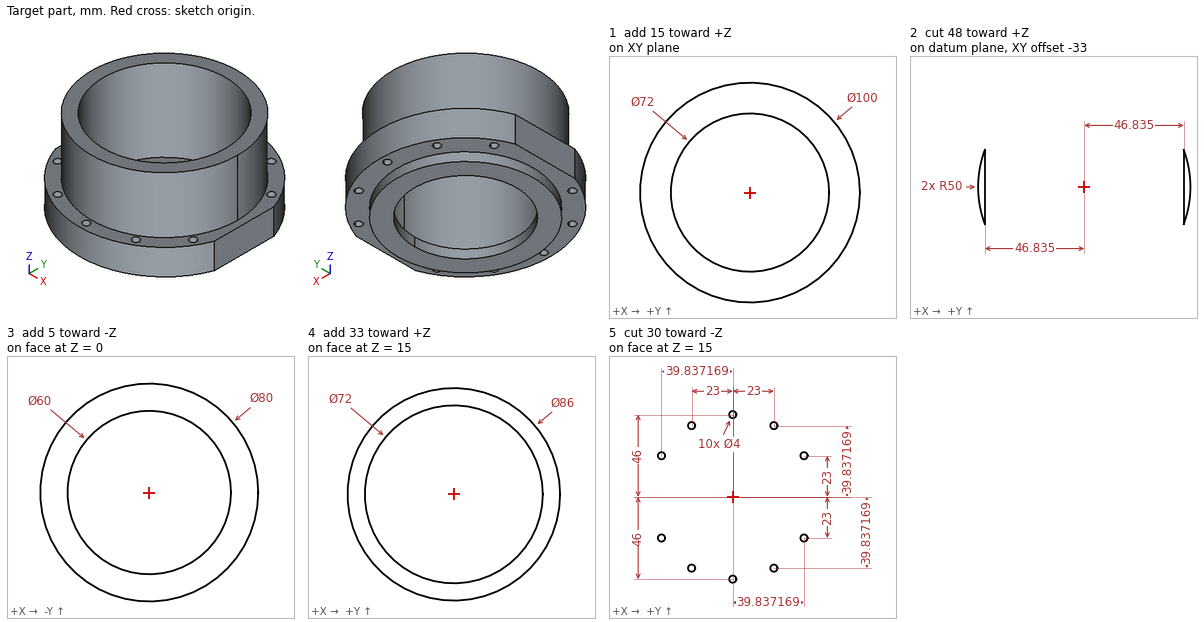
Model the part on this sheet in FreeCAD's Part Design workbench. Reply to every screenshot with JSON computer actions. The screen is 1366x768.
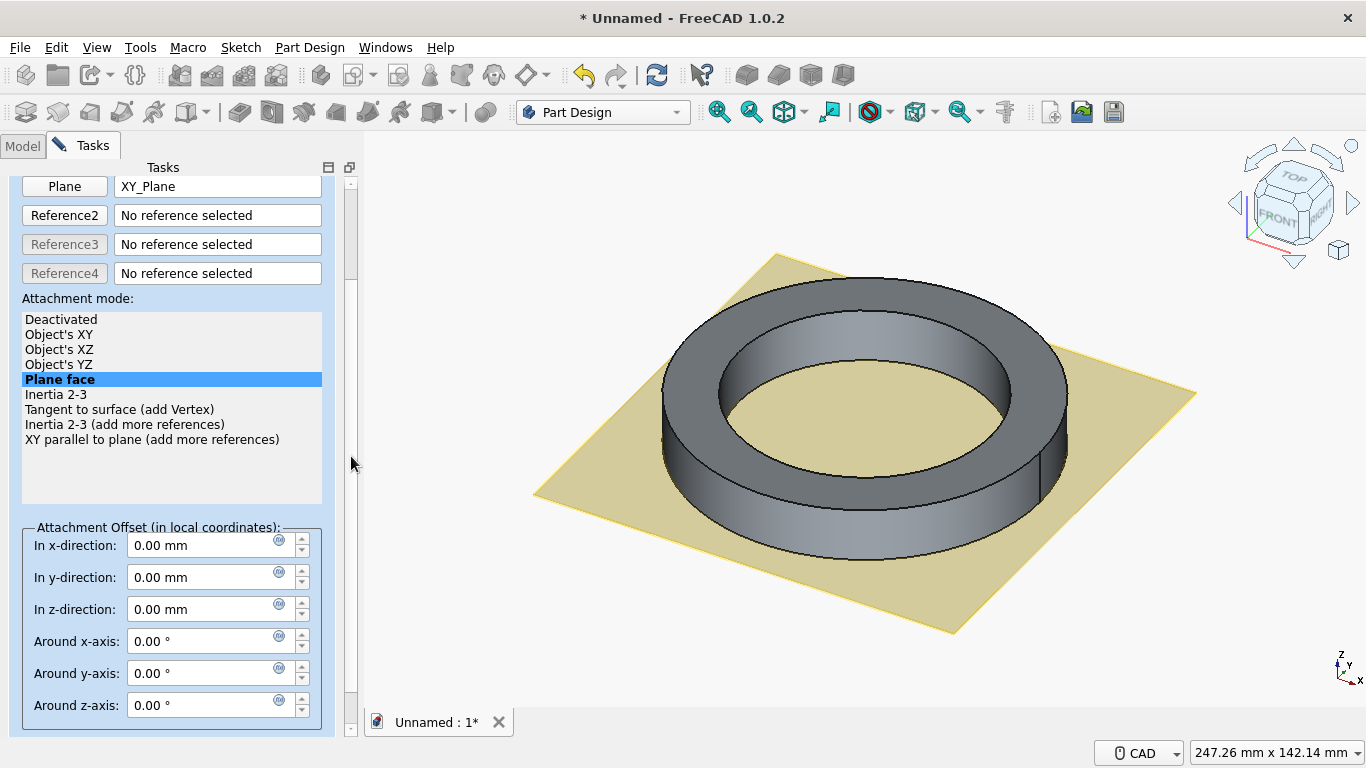
{"action": "triple_click", "coordinate": [210, 609]}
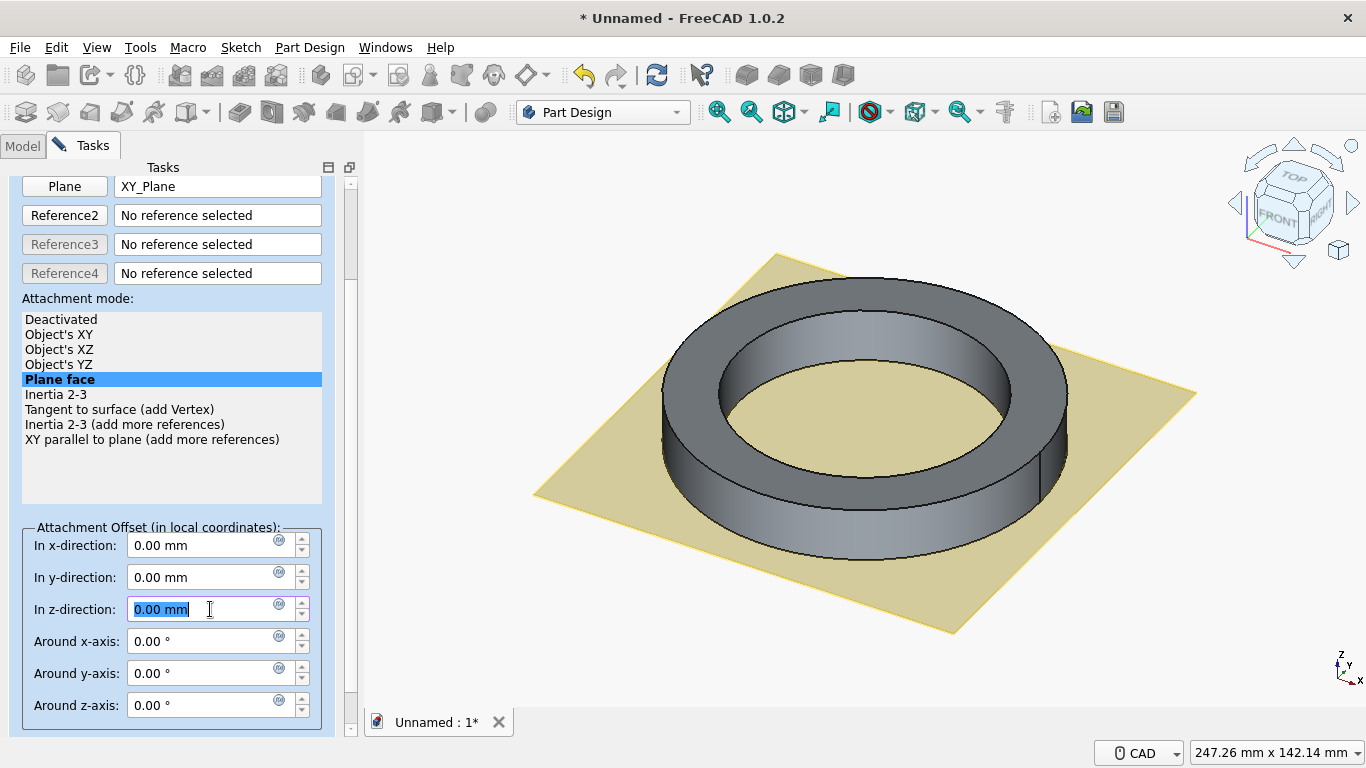
{"action": "type", "text": "-33"}
{"action": "key", "text": "Tab"}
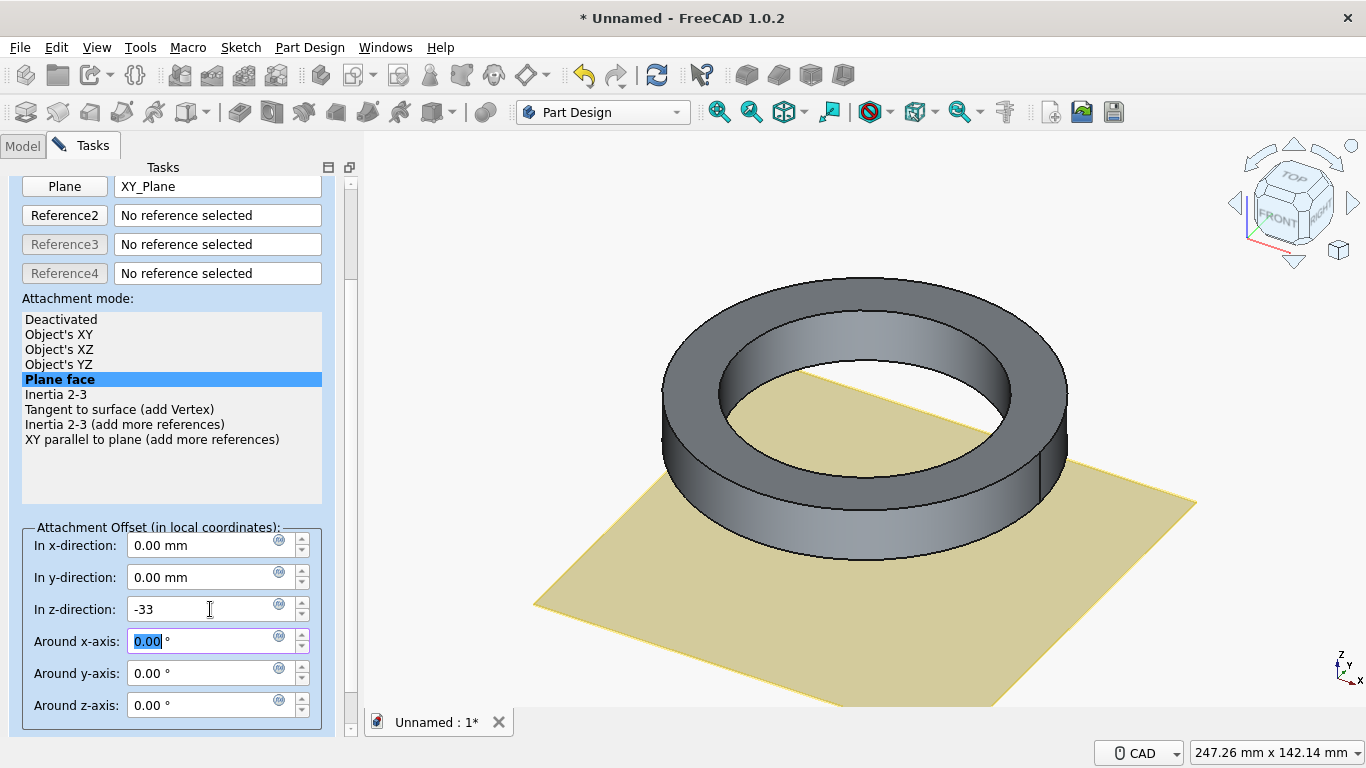
{"action": "scroll", "coordinate": [351, 456], "scroll_direction": "up", "scroll_amount": 3}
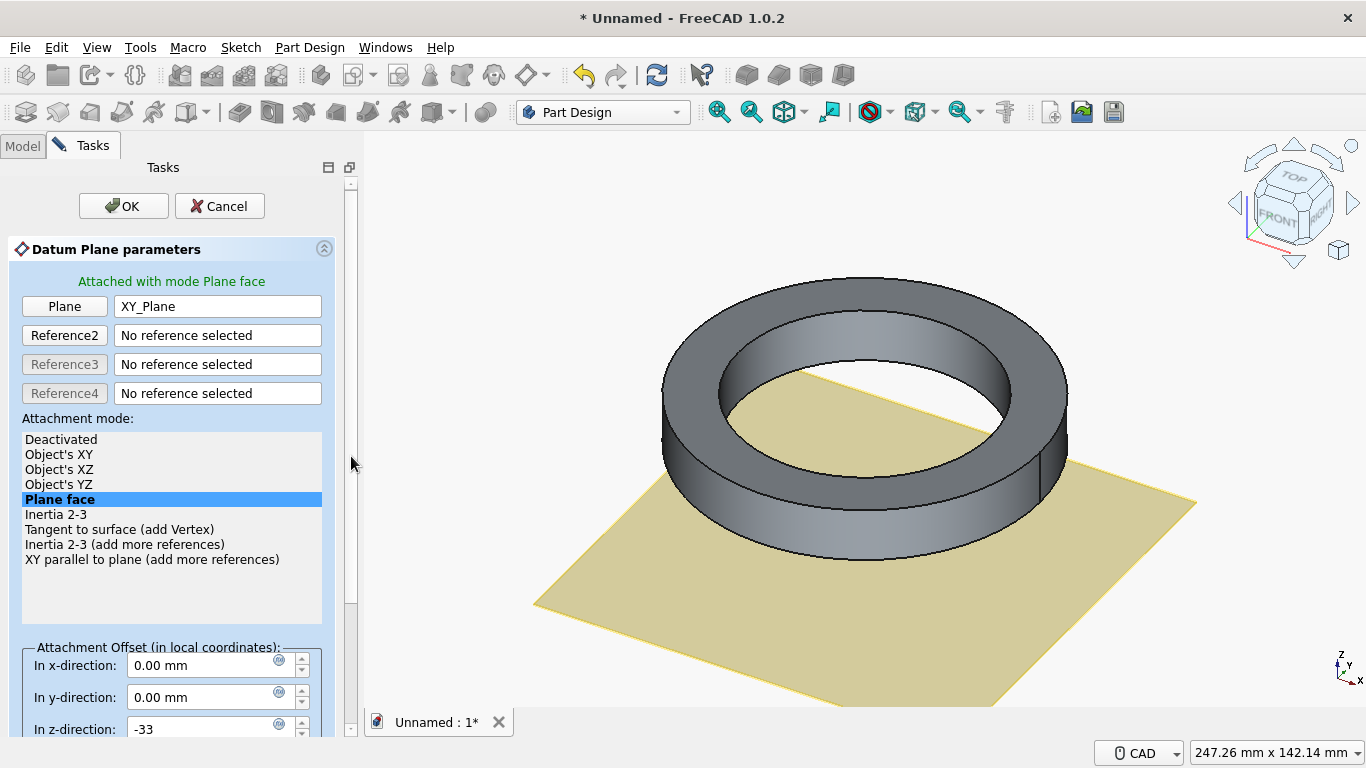
{"action": "left_click", "coordinate": [124, 206]}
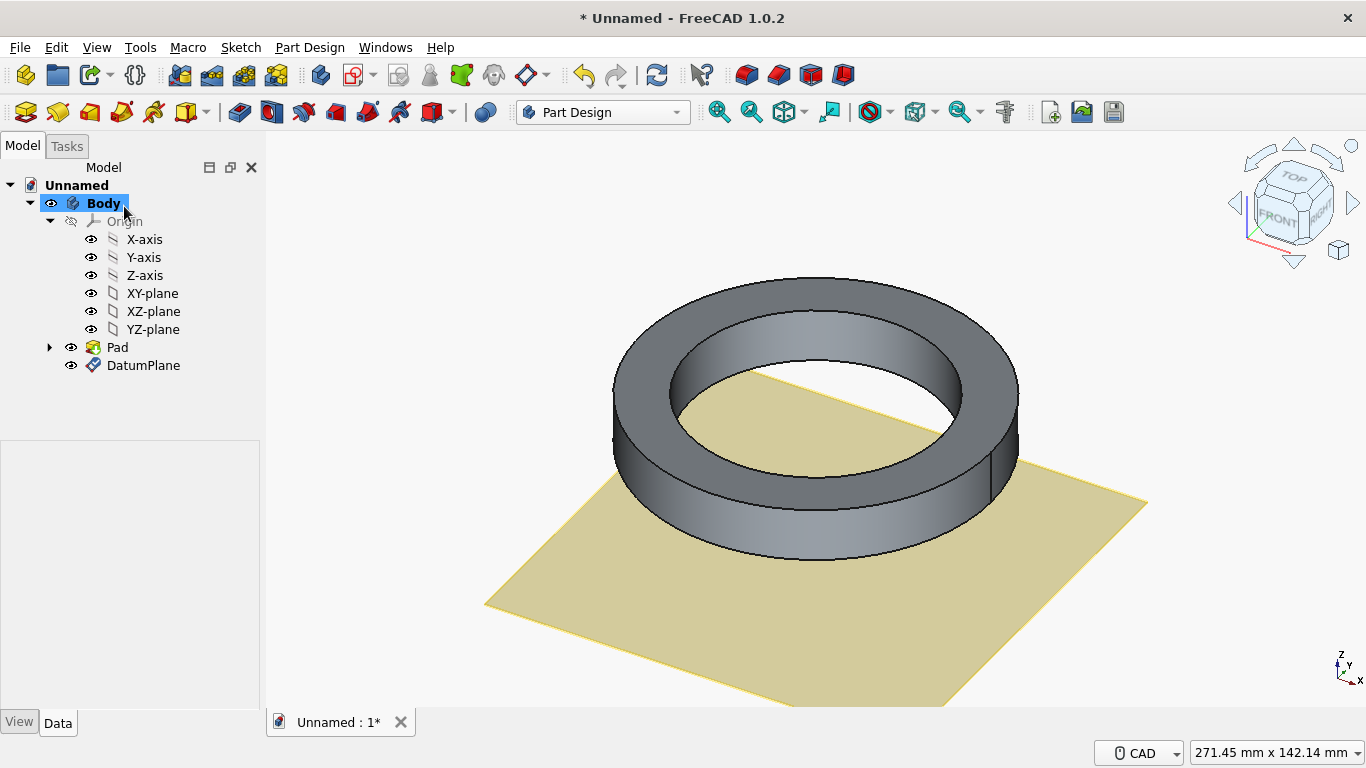
{"action": "left_click", "coordinate": [116, 365]}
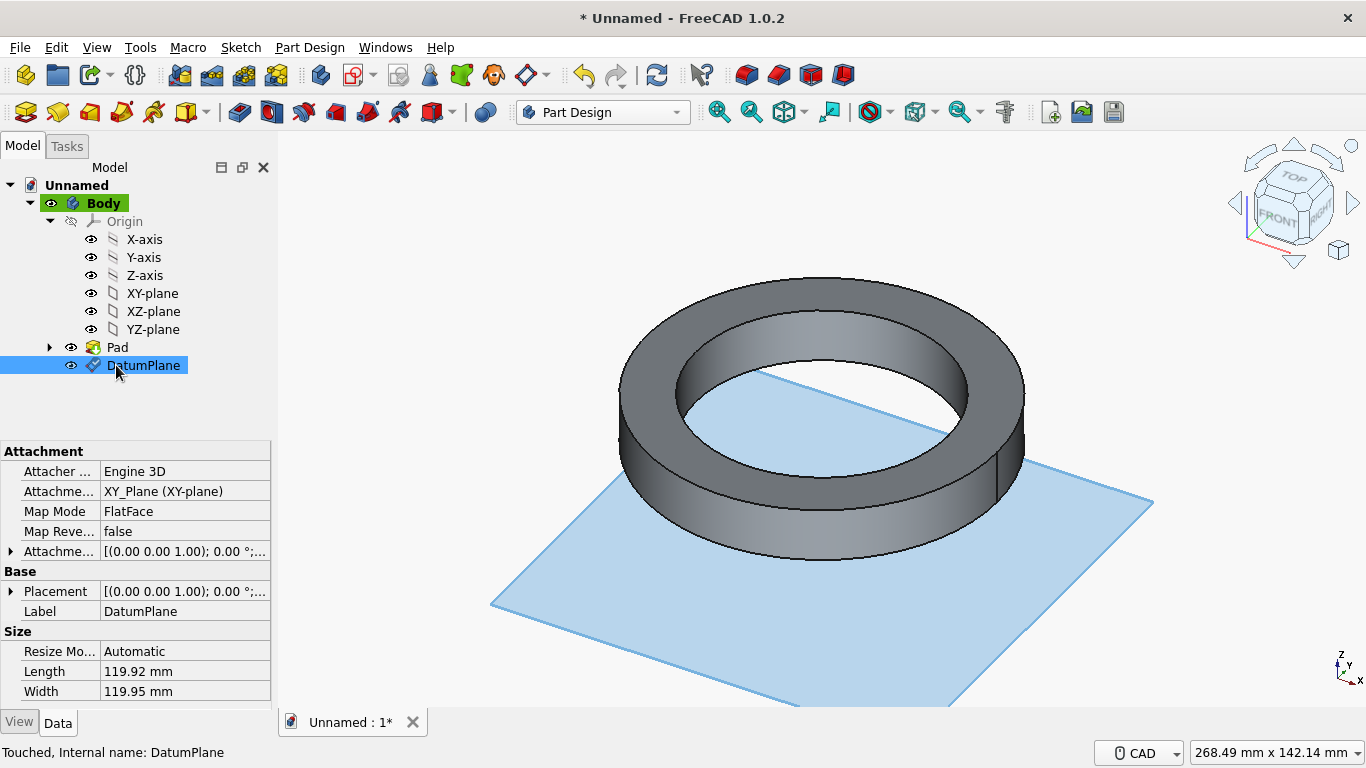
{"action": "left_click", "coordinate": [354, 76]}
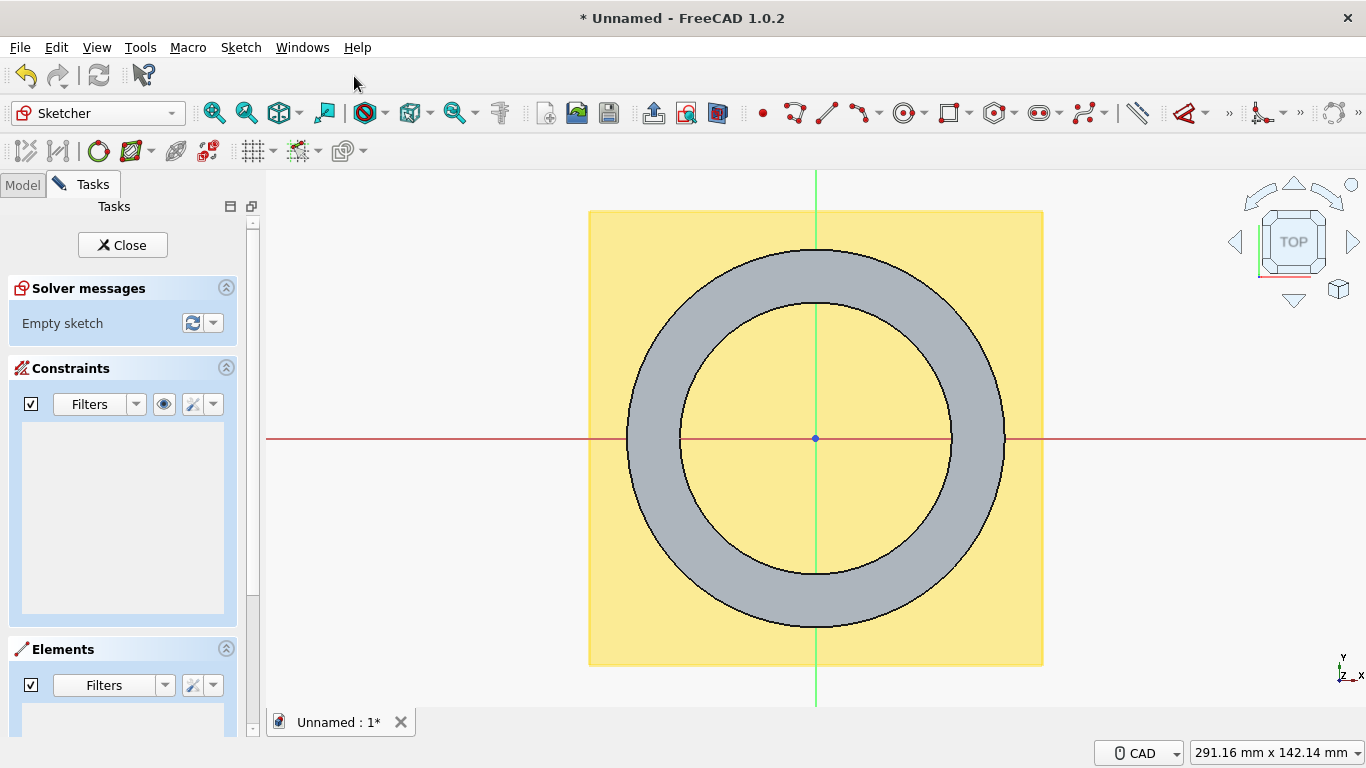
{"action": "left_click", "coordinate": [718, 114]}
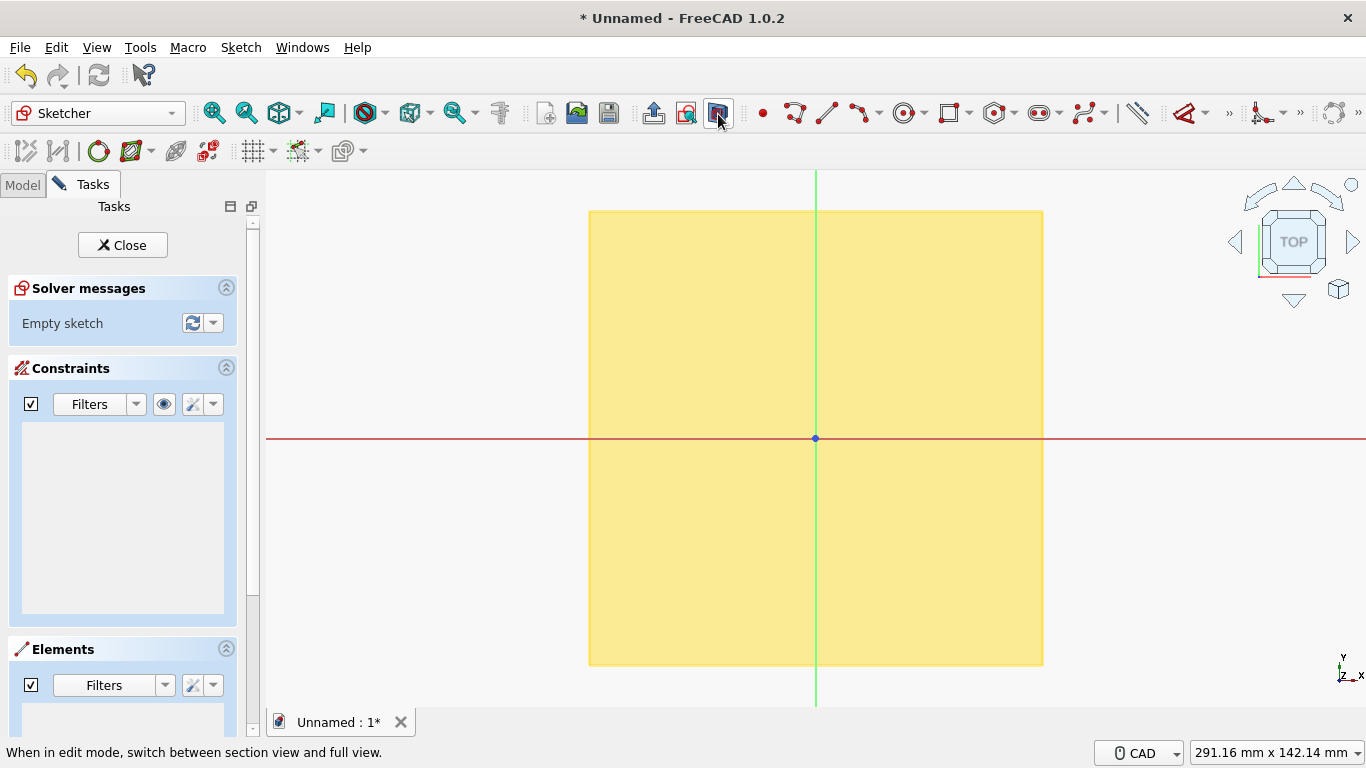
{"action": "scroll", "coordinate": [899, 438], "scroll_direction": "up", "scroll_amount": 3}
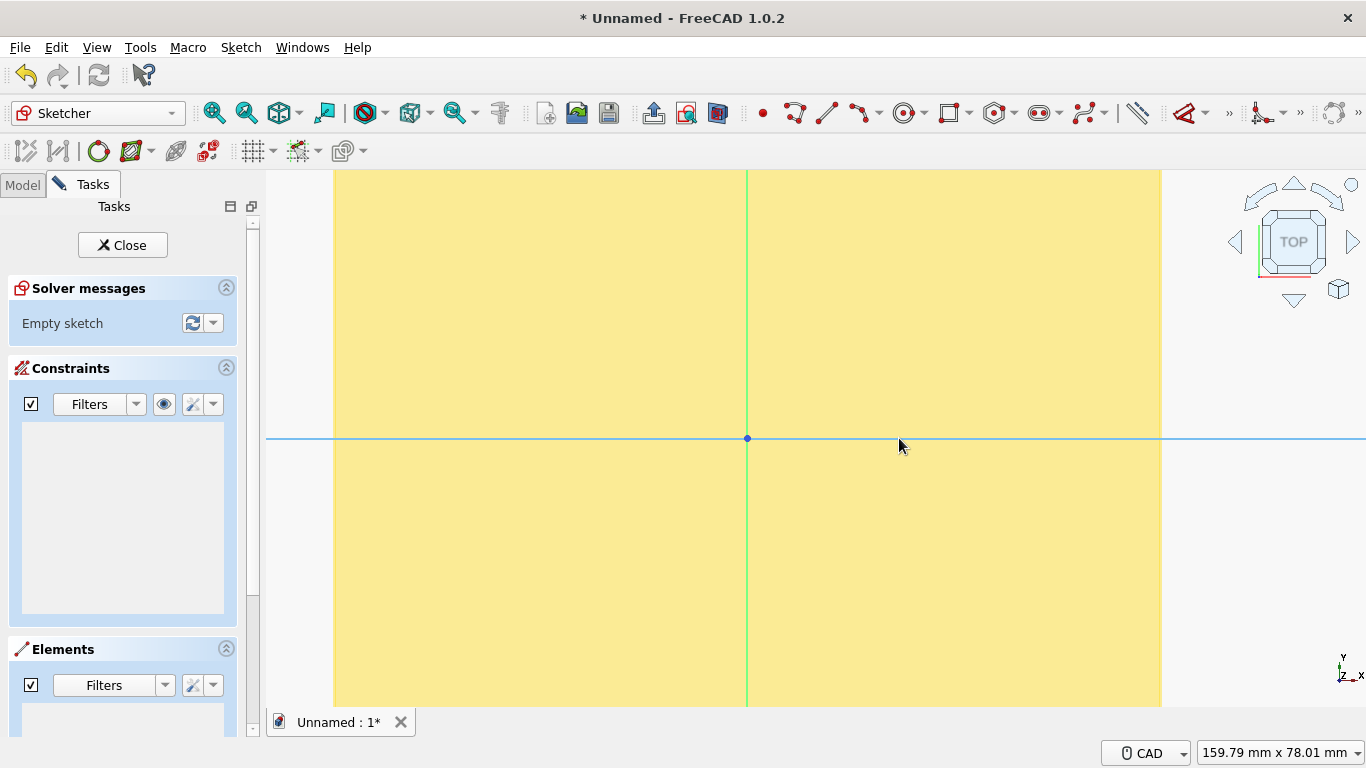
{"action": "left_click", "coordinate": [828, 114]}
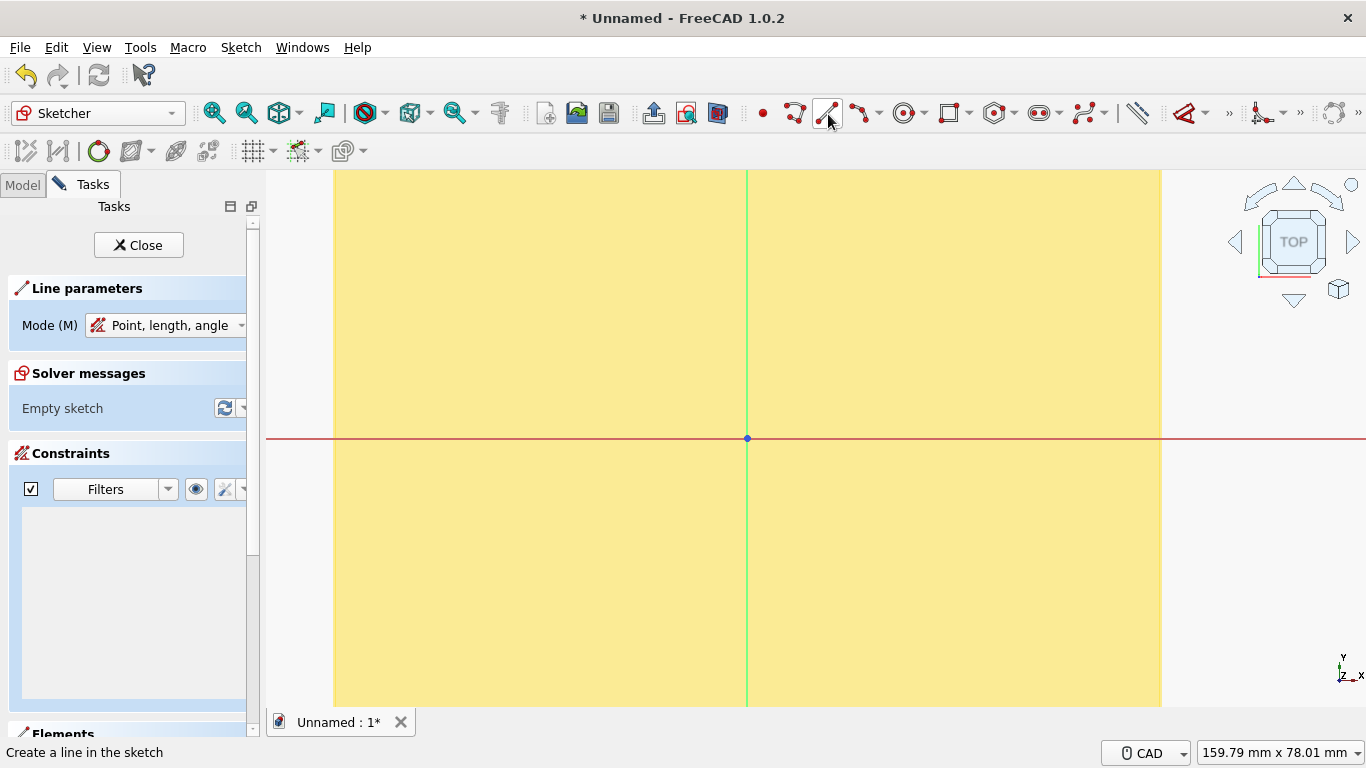
{"action": "left_click", "coordinate": [425, 559]}
{"action": "left_click", "coordinate": [425, 318]}